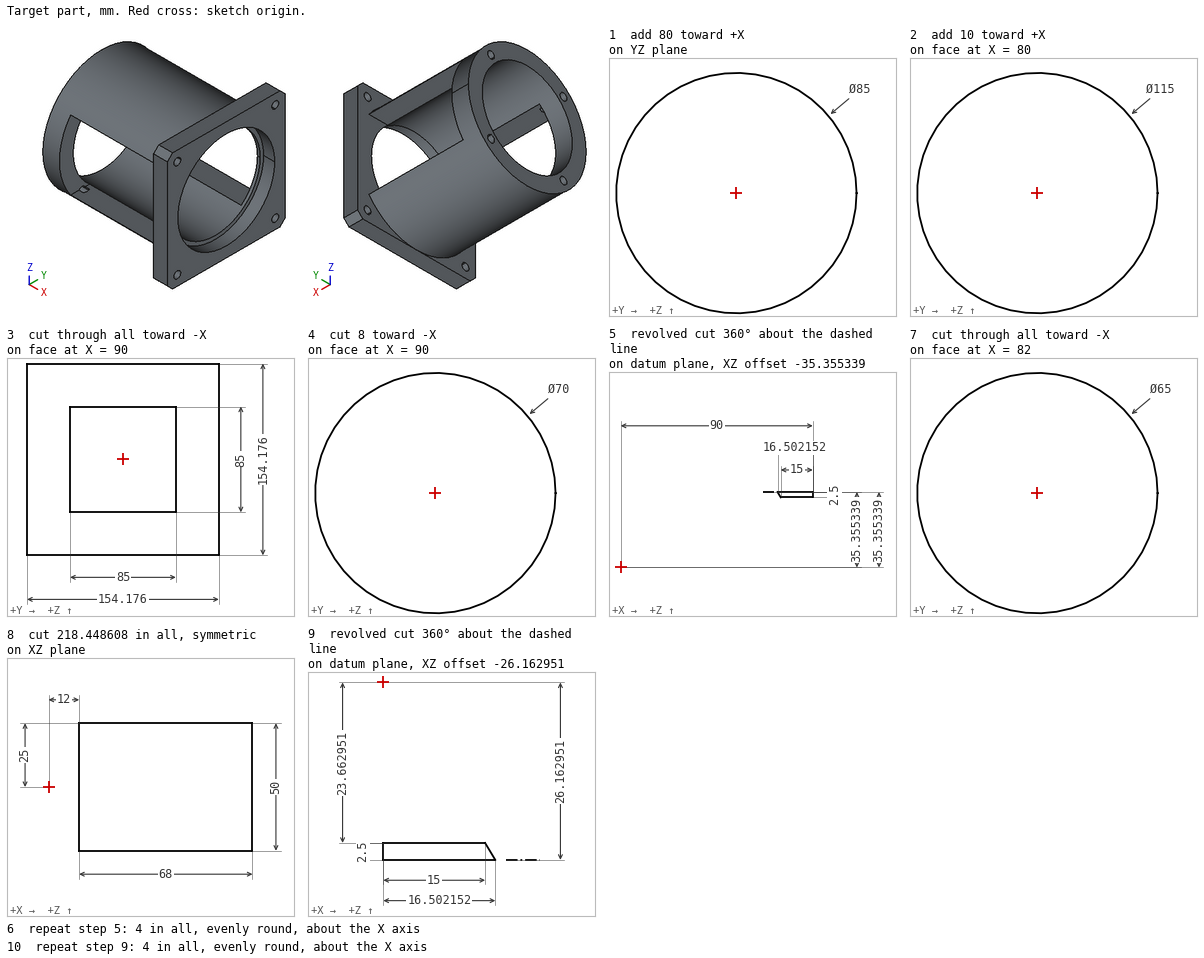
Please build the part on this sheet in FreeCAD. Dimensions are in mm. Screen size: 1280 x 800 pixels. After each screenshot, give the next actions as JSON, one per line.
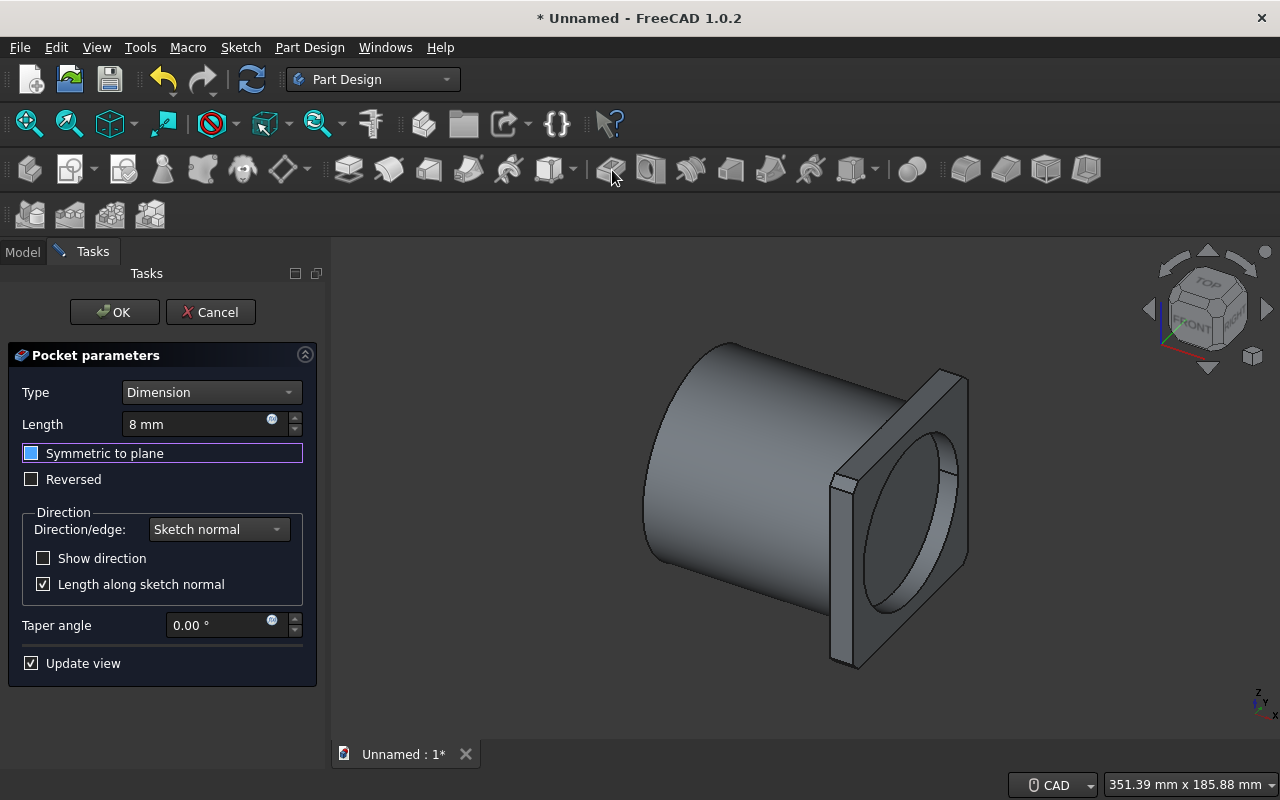
{"action": "left_click", "coordinate": [115, 312]}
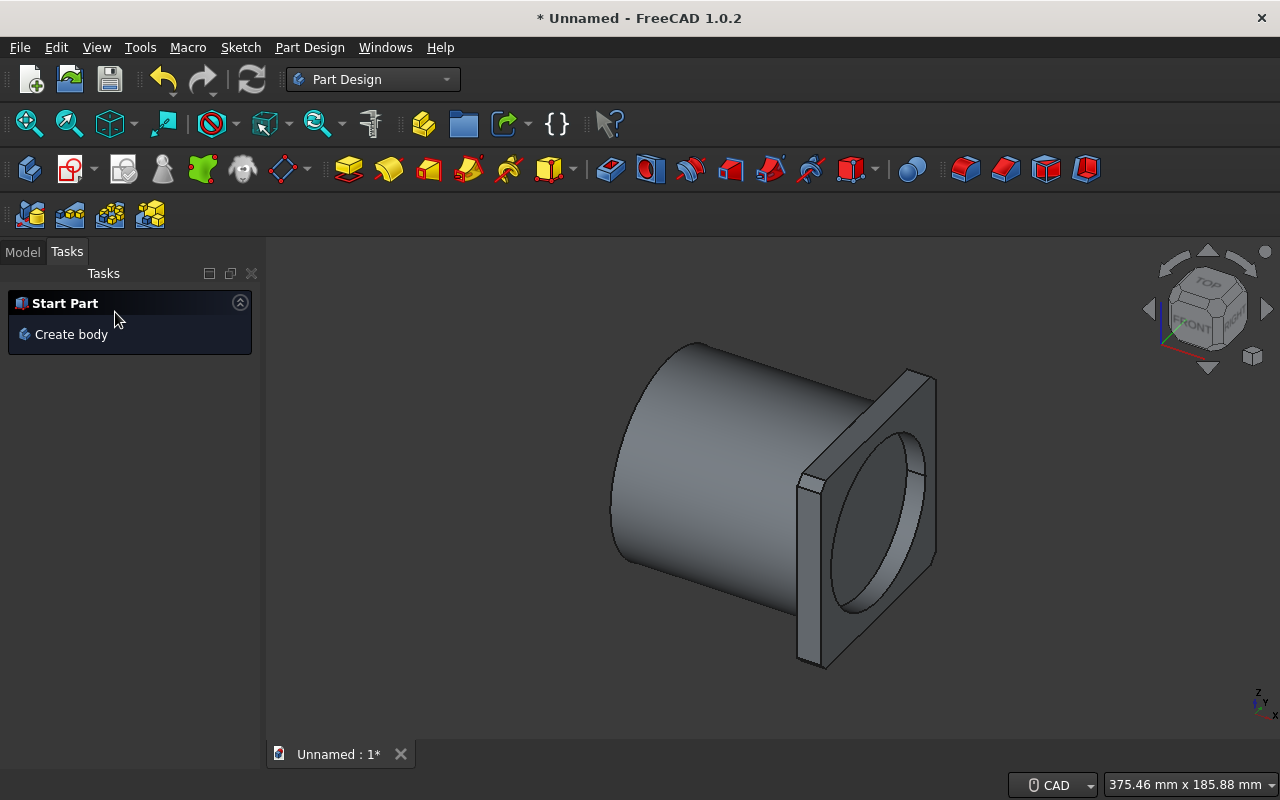
{"action": "left_click", "coordinate": [23, 251]}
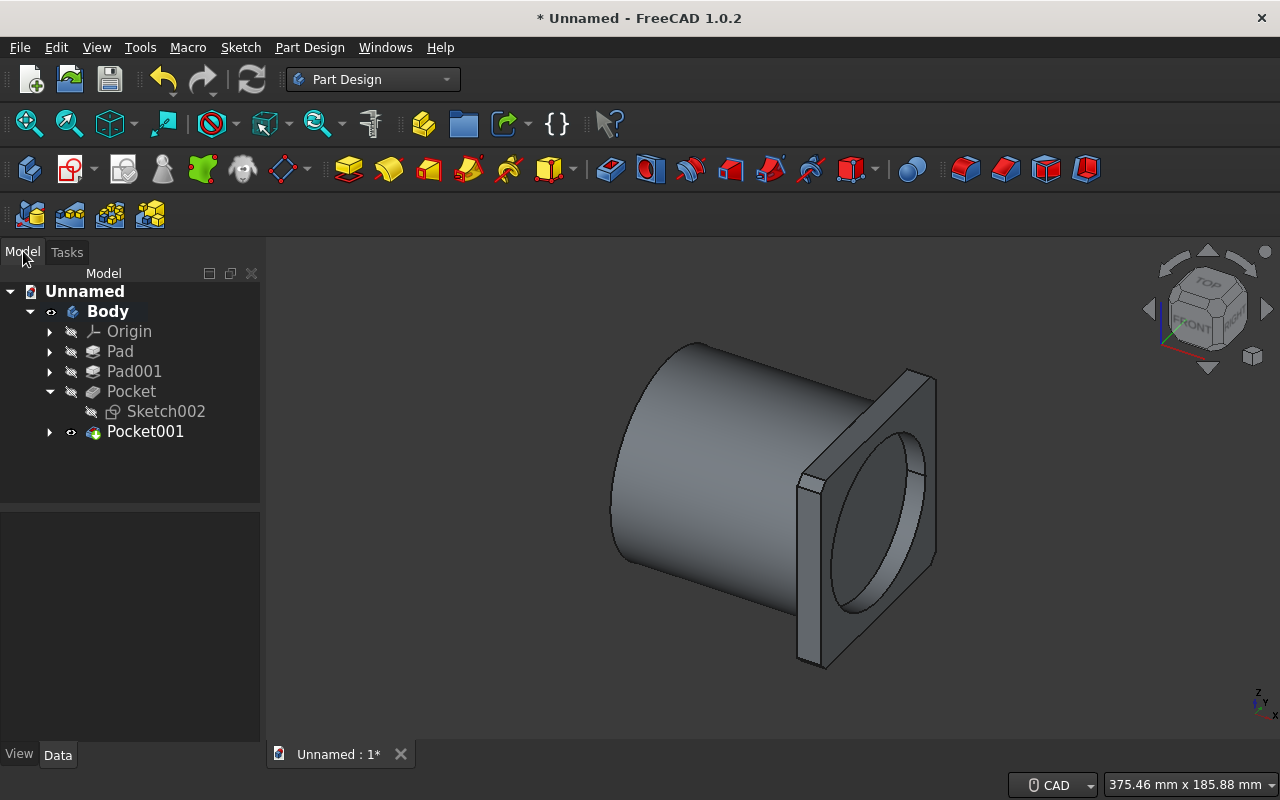
{"action": "left_click", "coordinate": [50, 332]}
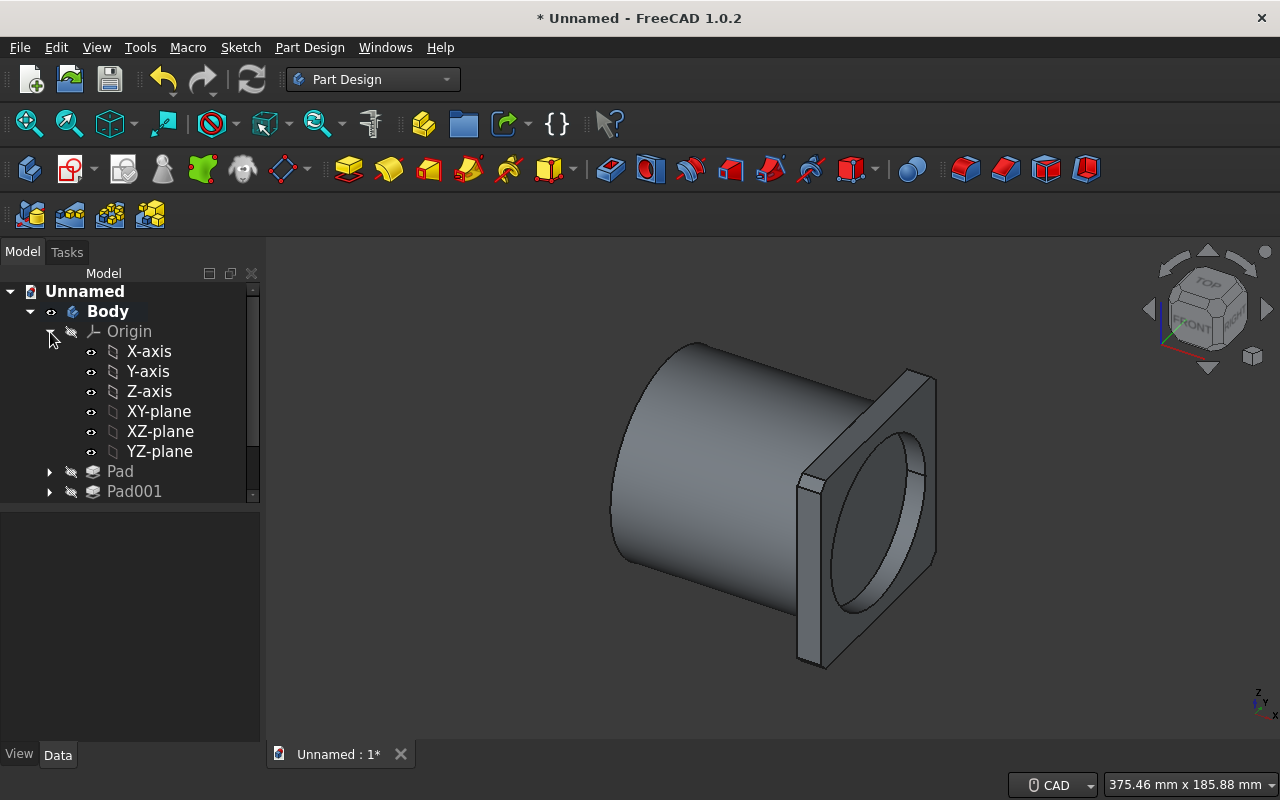
{"action": "left_click", "coordinate": [136, 432]}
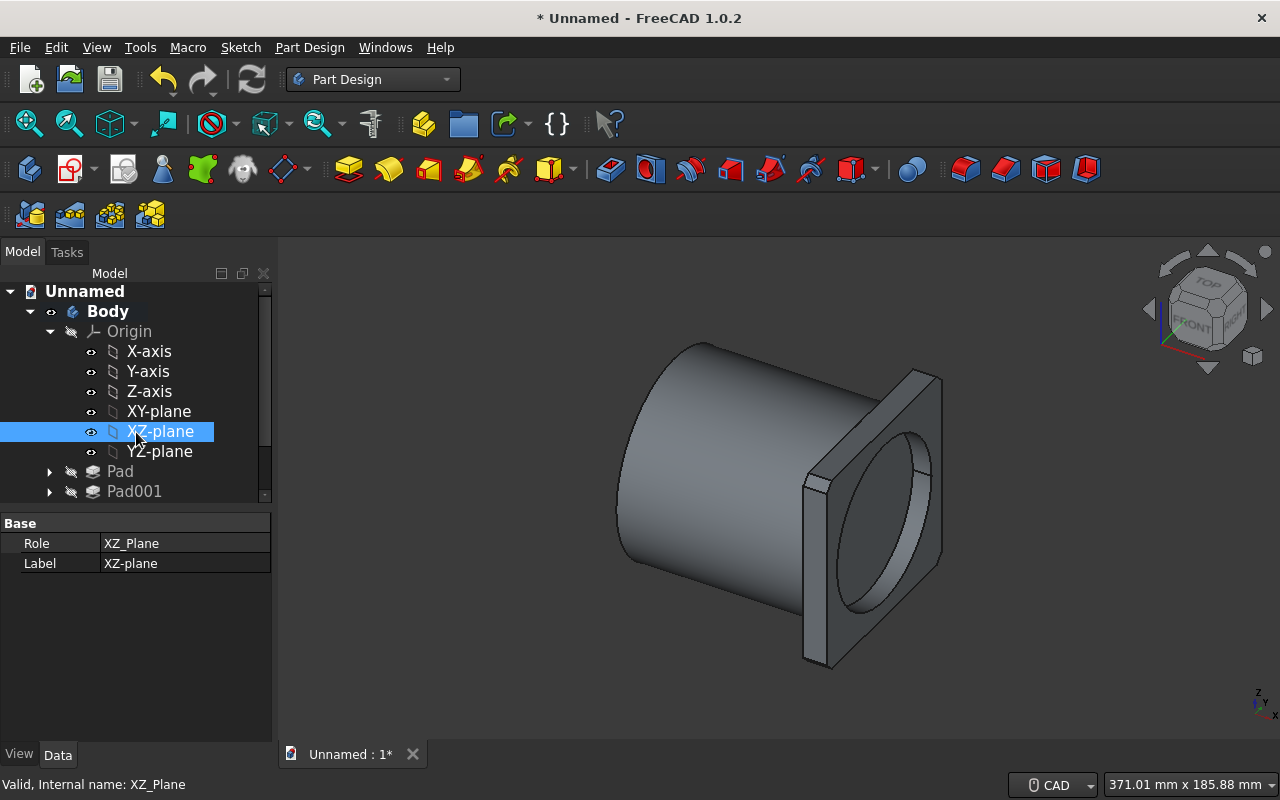
{"action": "left_click", "coordinate": [284, 170]}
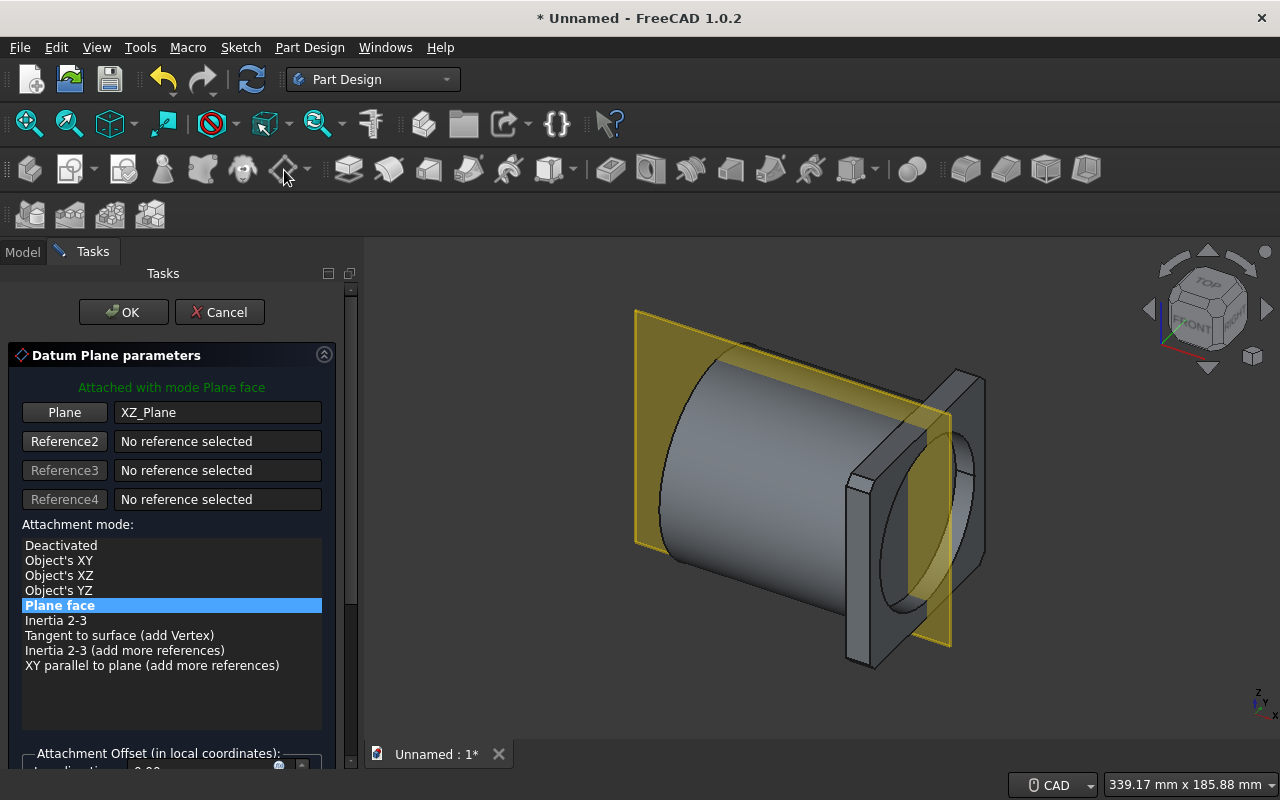
{"action": "scroll", "coordinate": [351, 526], "scroll_direction": "down", "scroll_amount": 3}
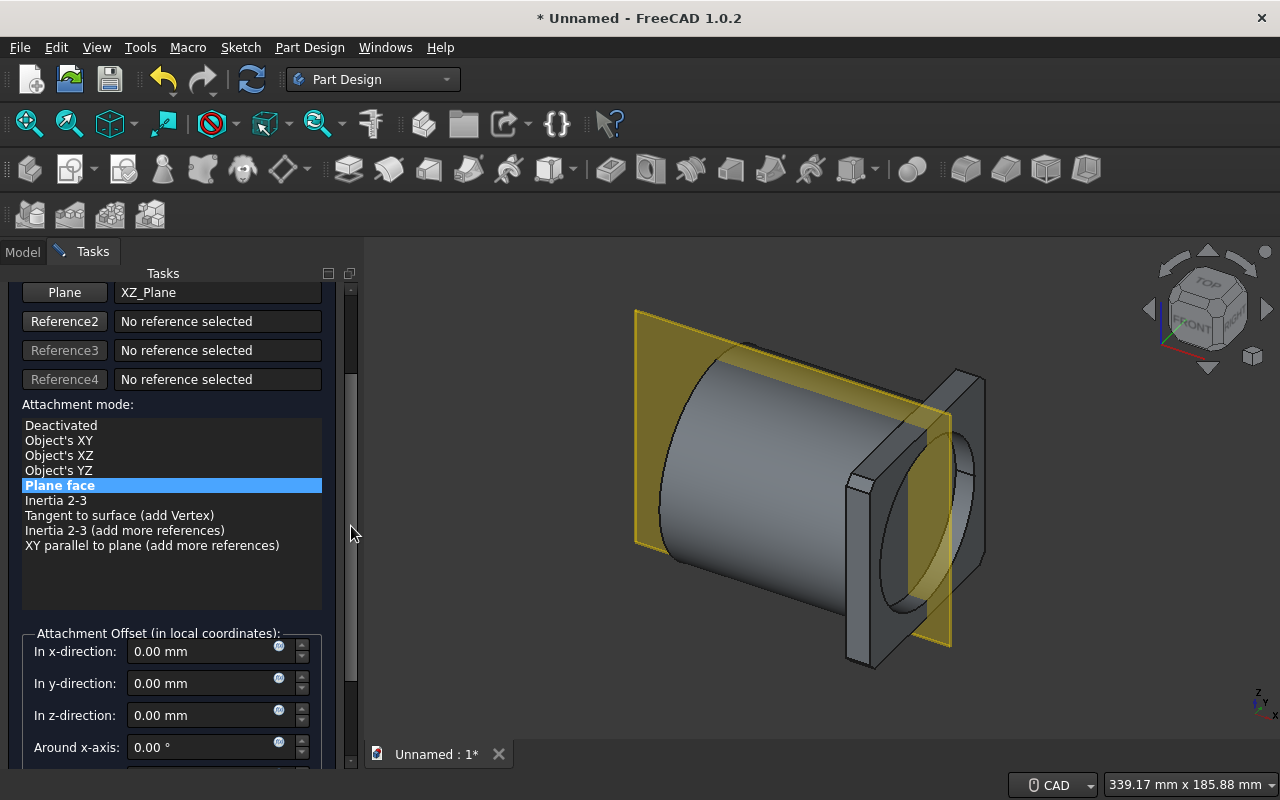
{"action": "triple_click", "coordinate": [210, 655]}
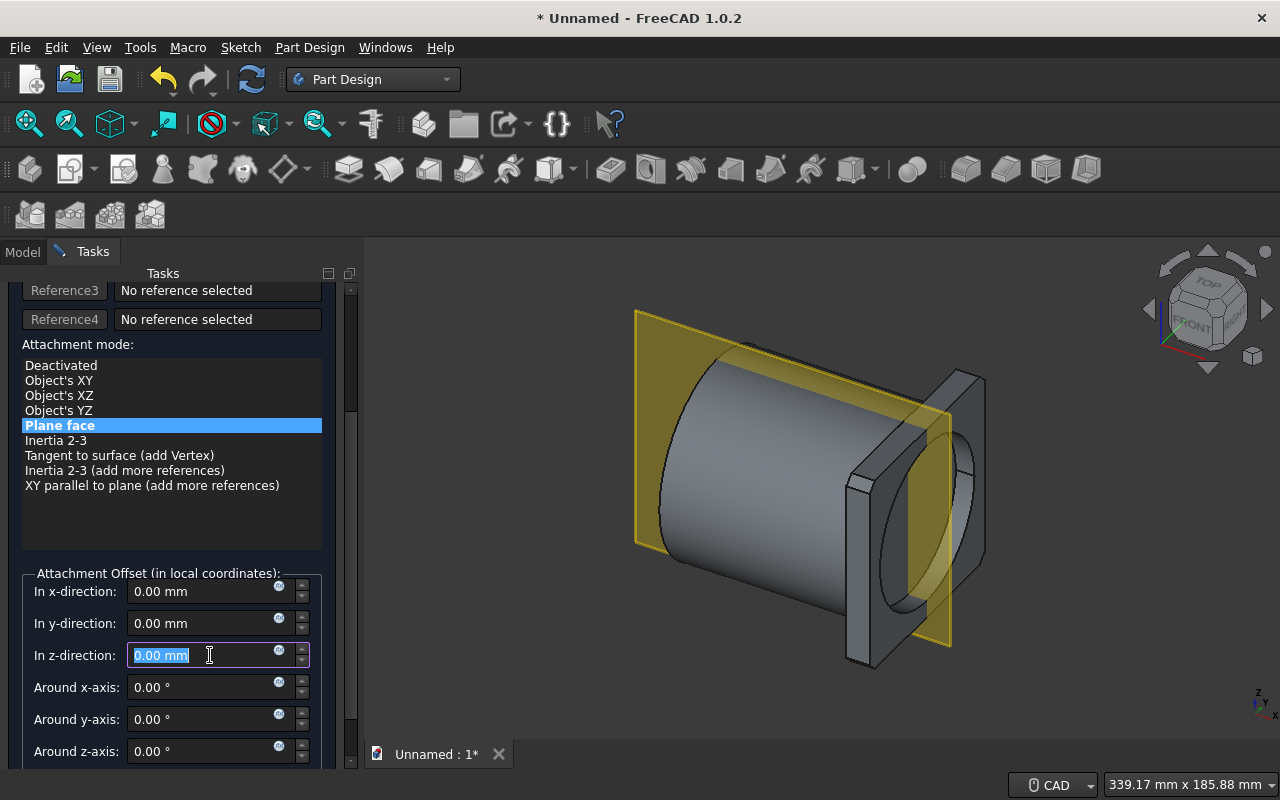
{"action": "type", "text": "-35.355339"}
{"action": "key", "text": "Tab"}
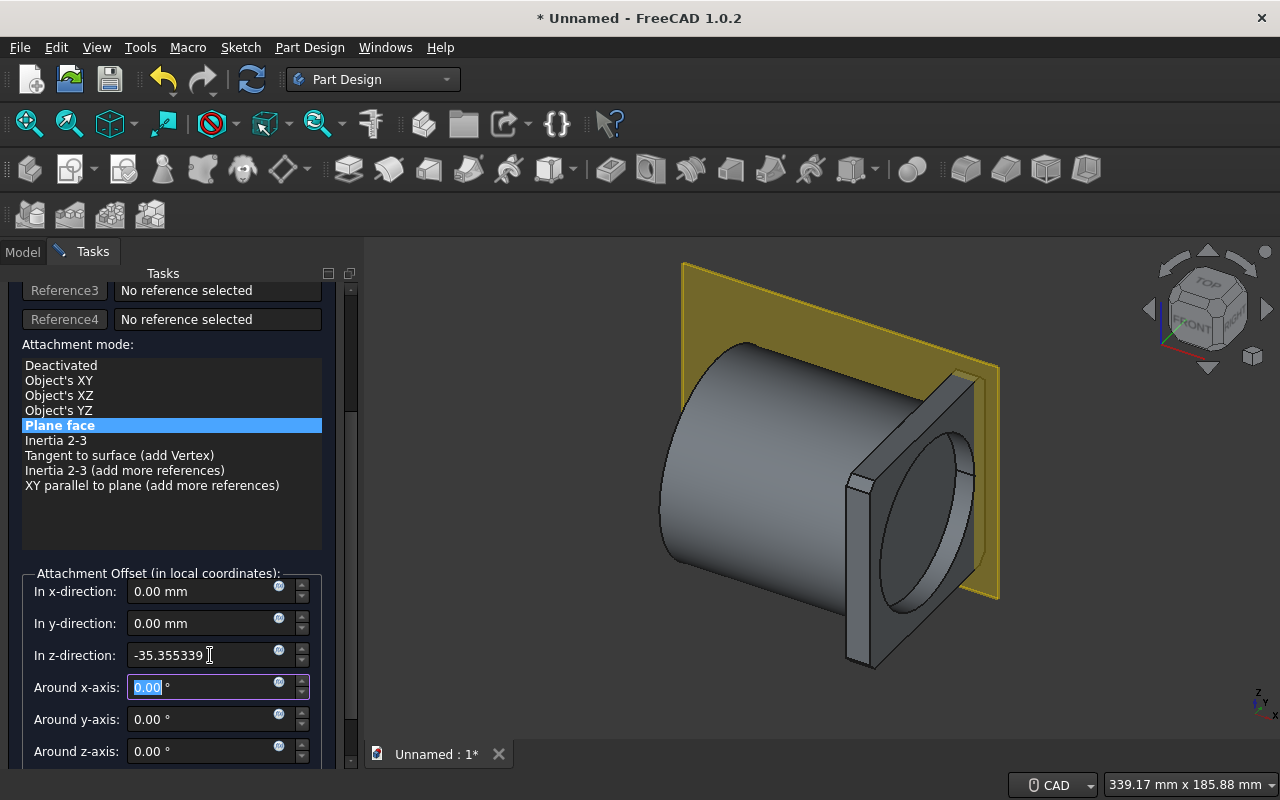
{"action": "scroll", "coordinate": [351, 526], "scroll_direction": "up", "scroll_amount": 4}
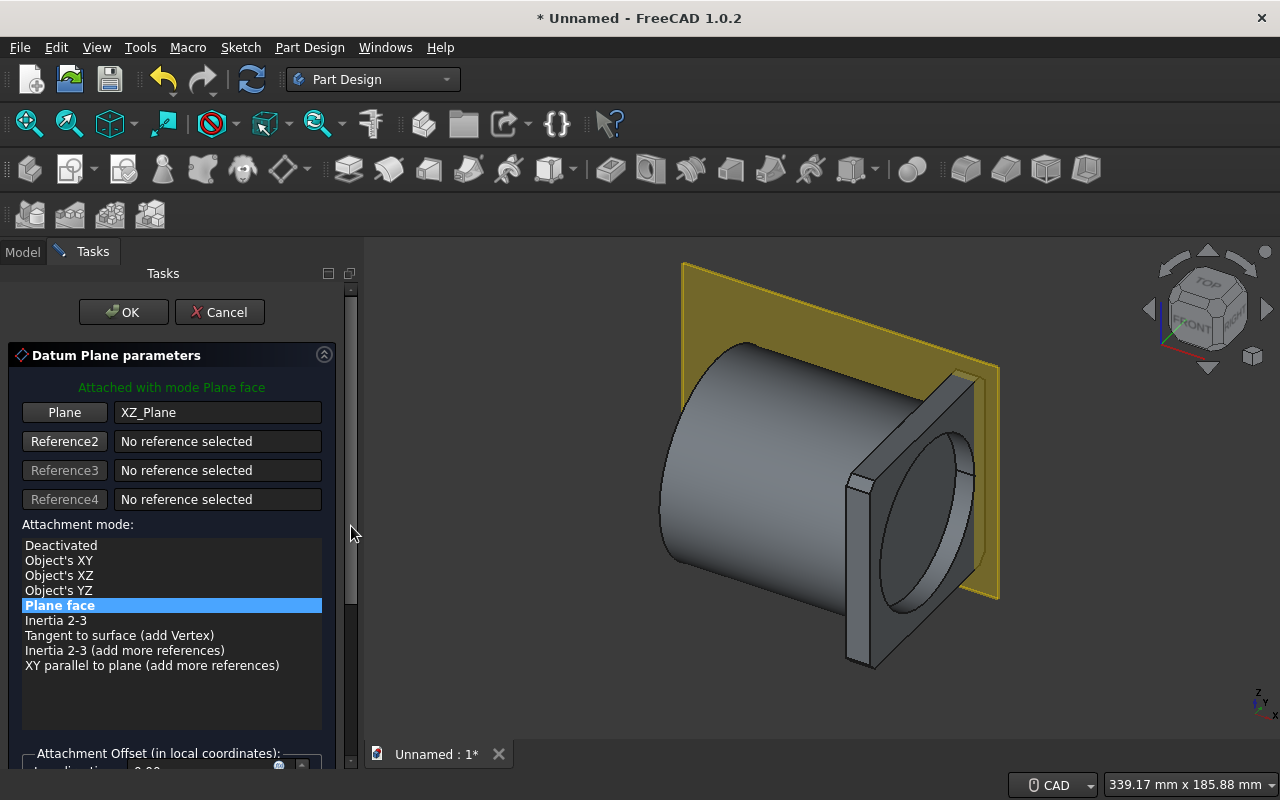
{"action": "left_click", "coordinate": [124, 312]}